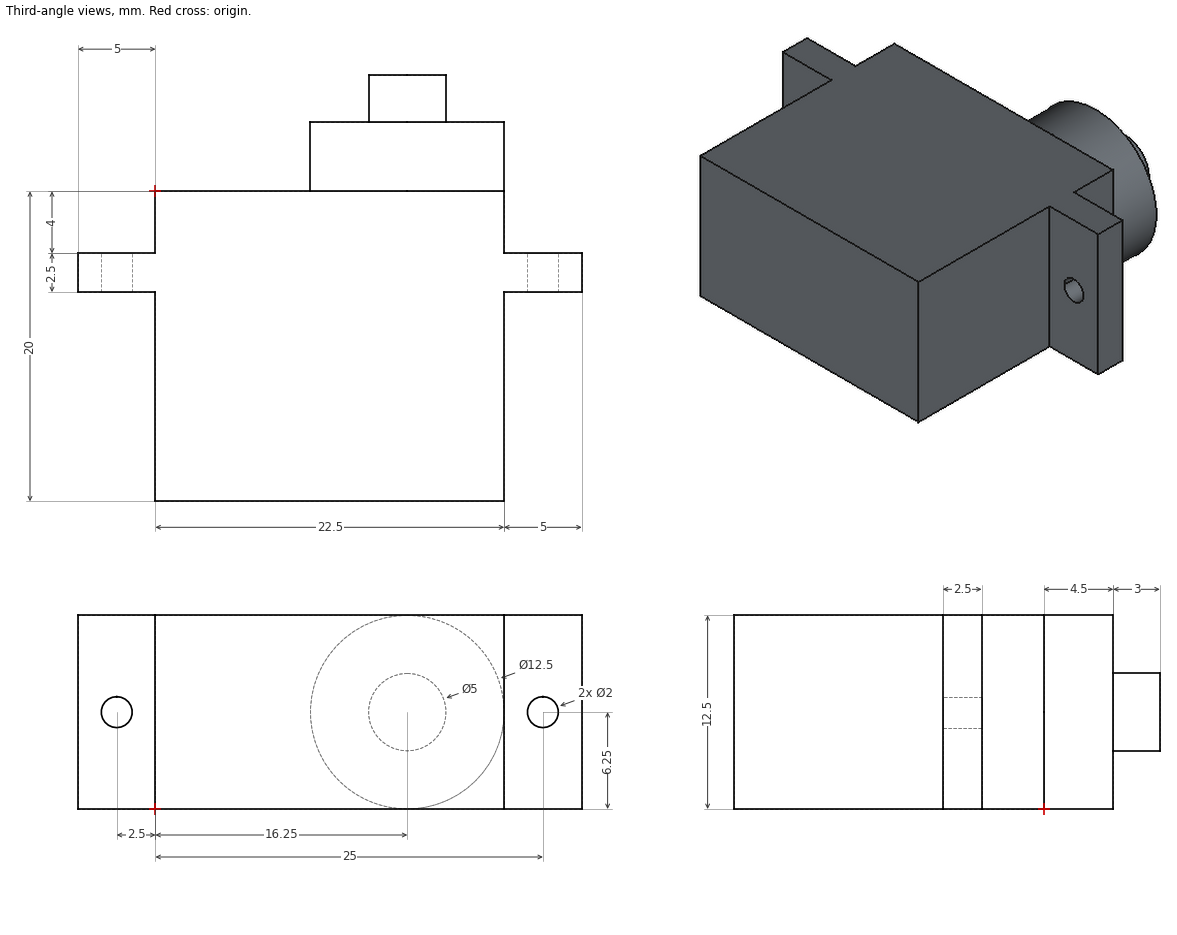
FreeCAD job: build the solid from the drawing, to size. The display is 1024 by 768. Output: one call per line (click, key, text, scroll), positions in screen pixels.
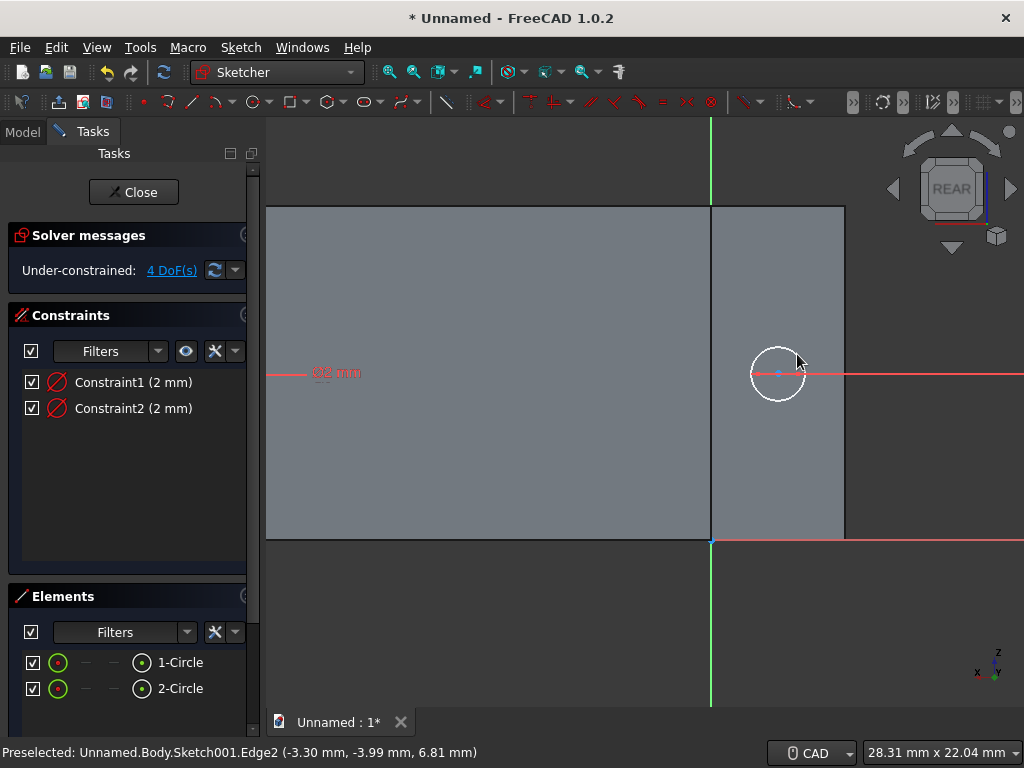
scroll(779, 374, down, 3)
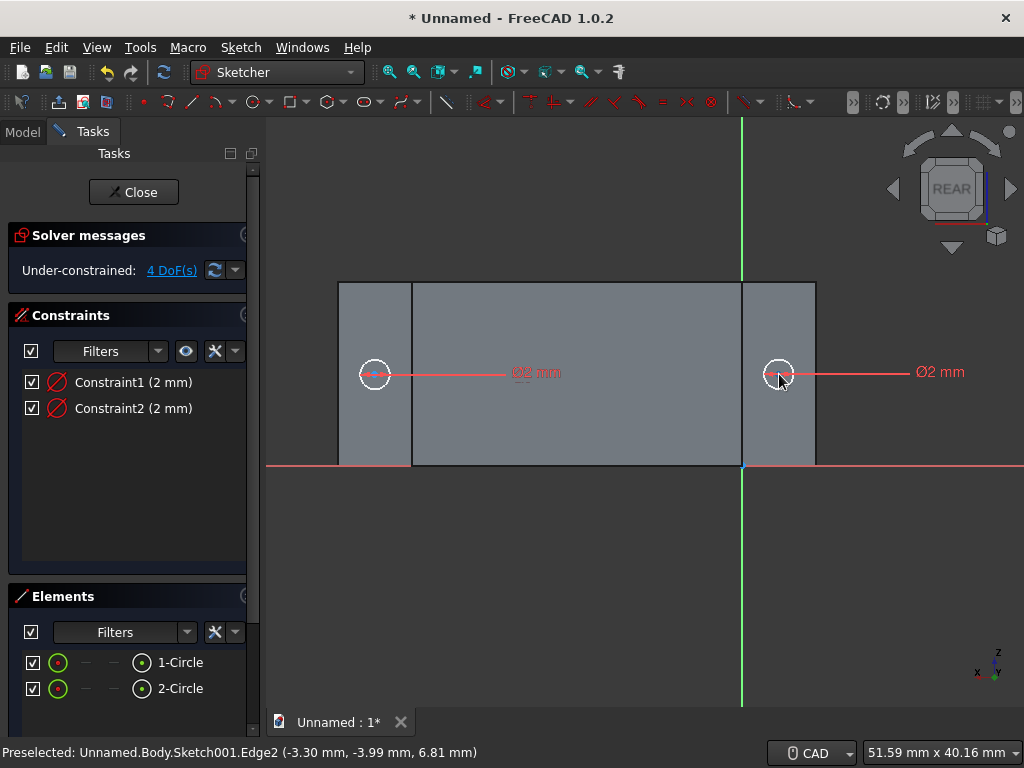
click(375, 375)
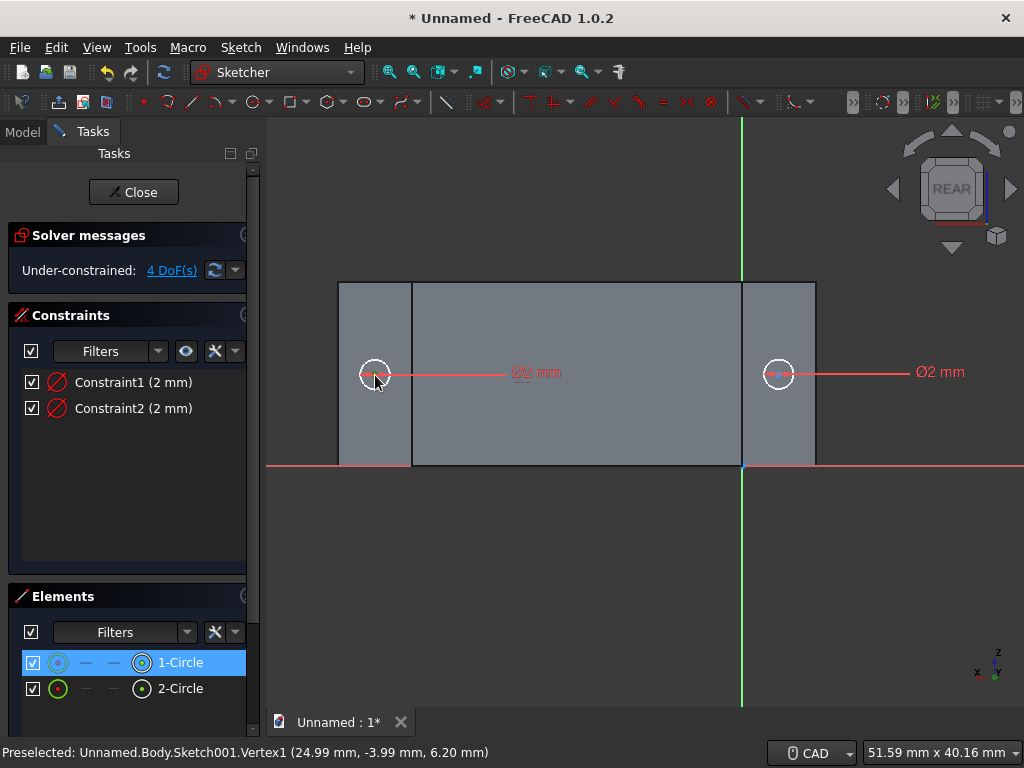
click(779, 374)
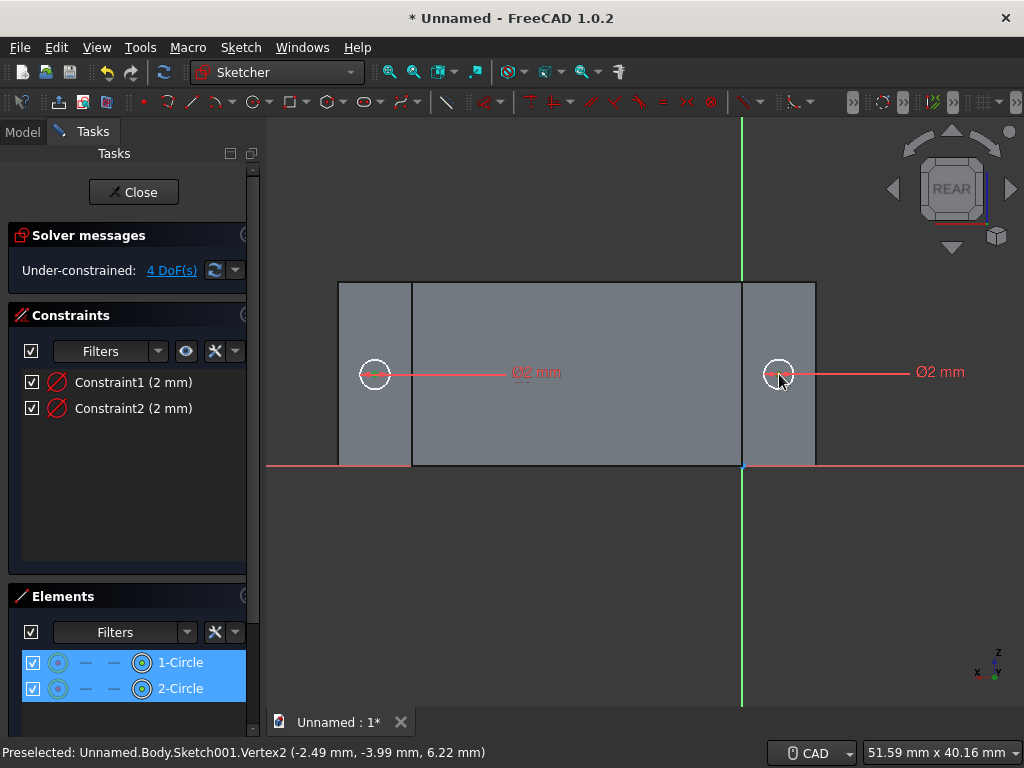
key(h)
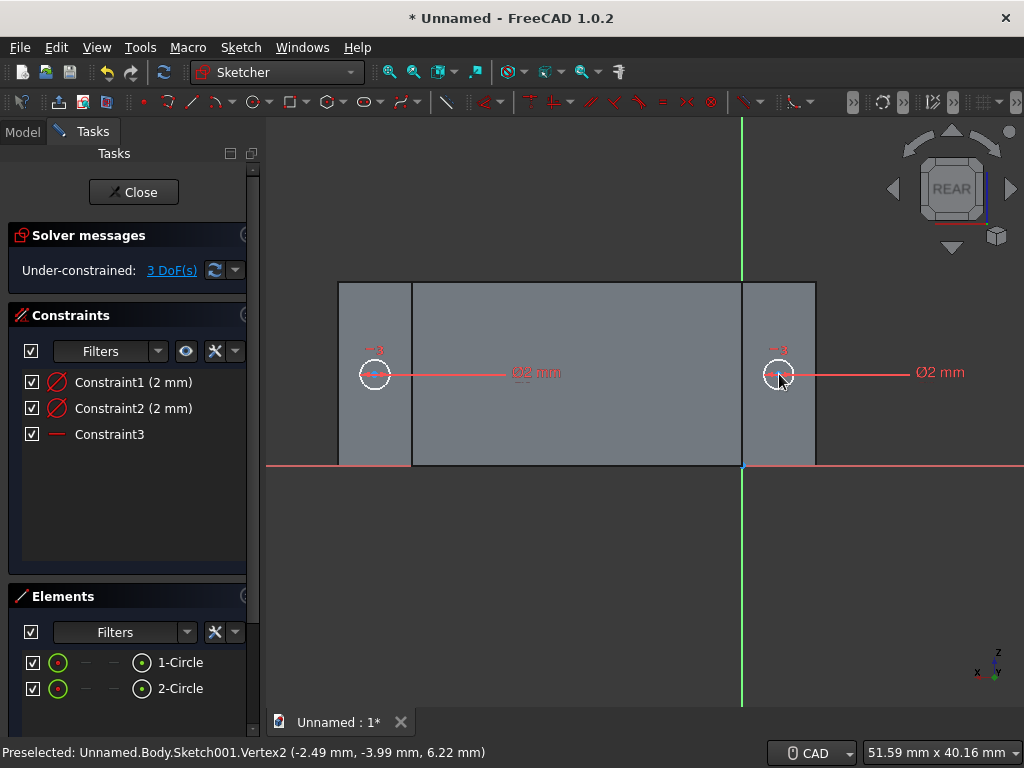
key(d)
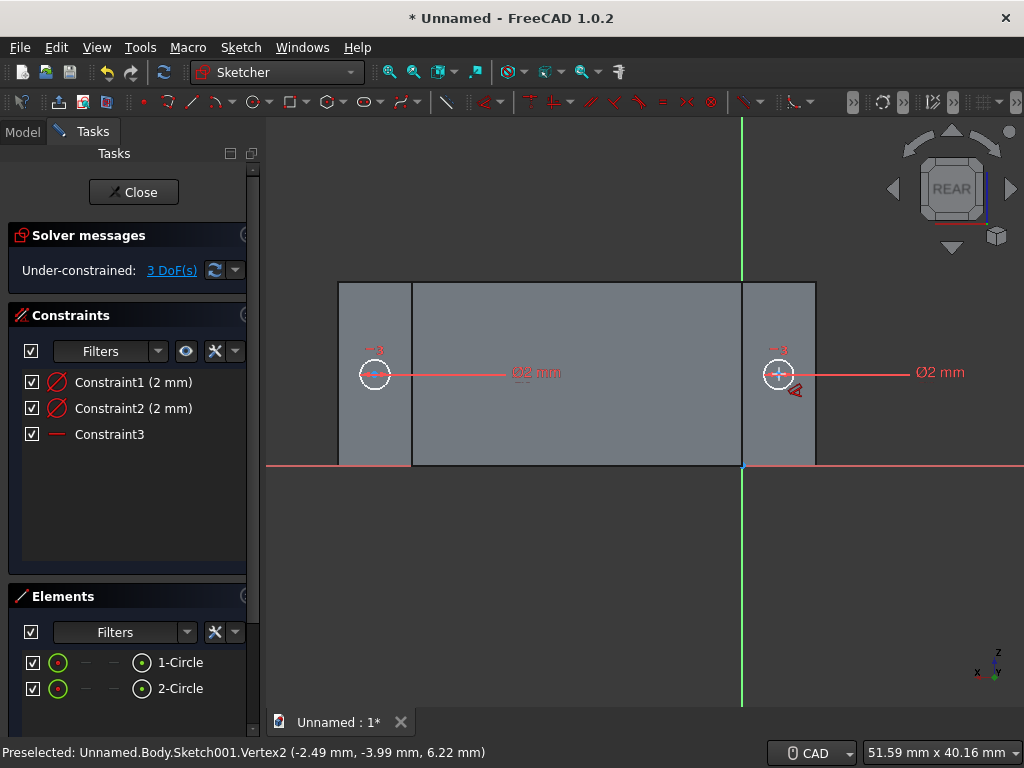
click(375, 375)
click(559, 500)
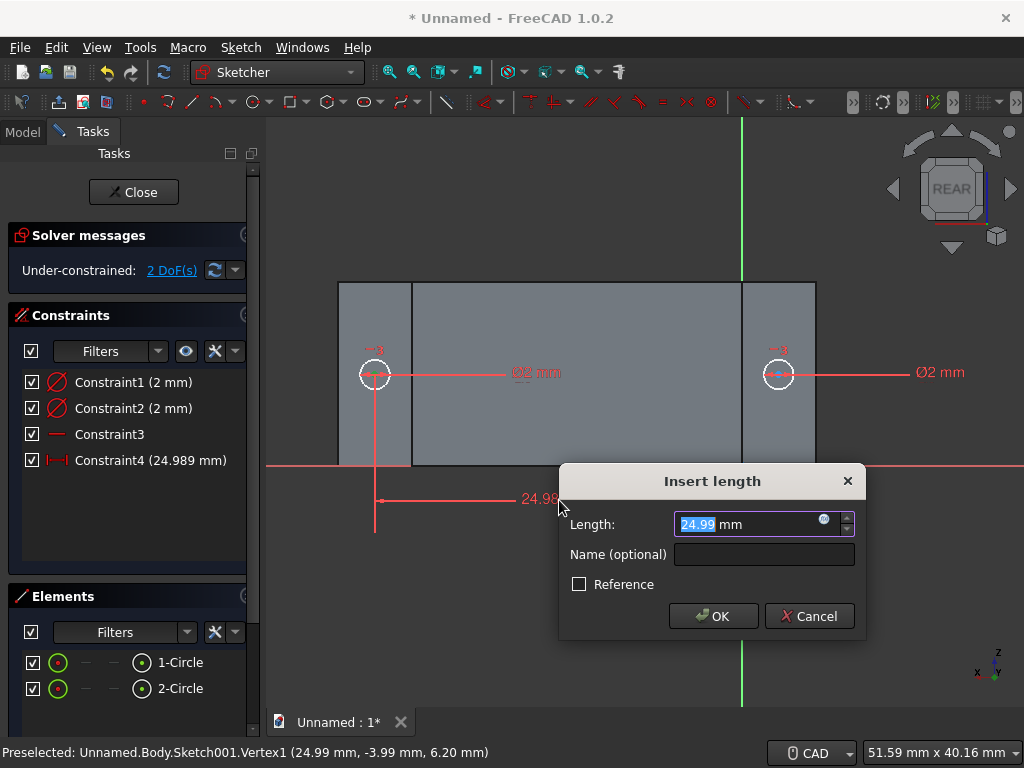
text(25)
key(Return)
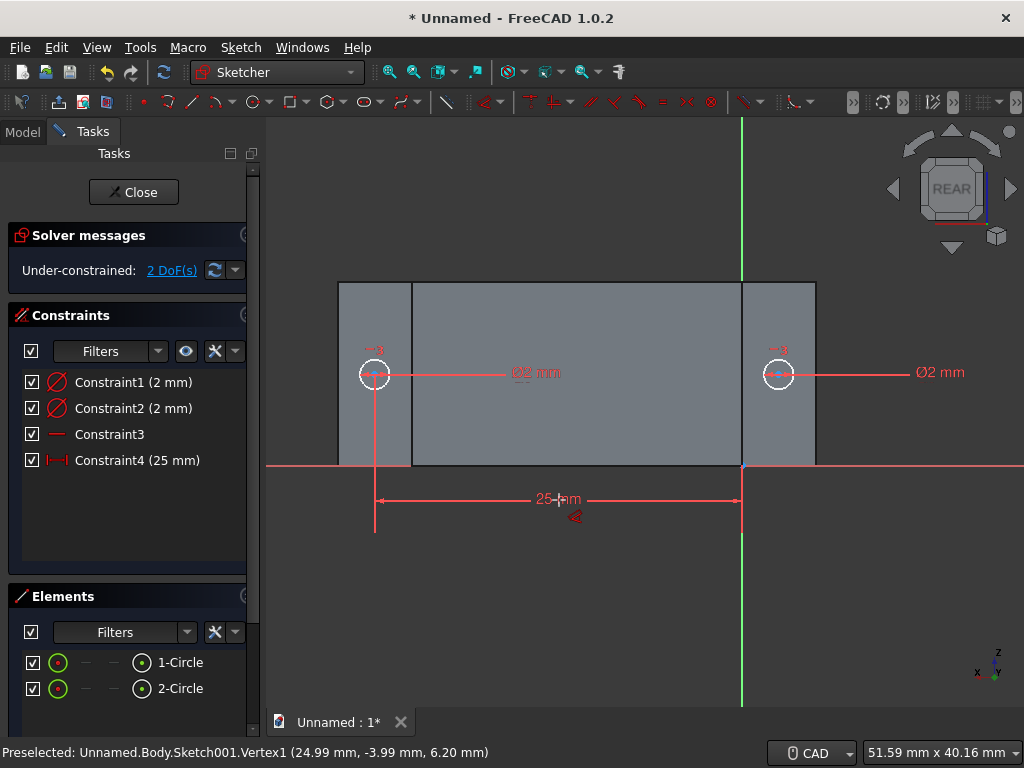
click(779, 375)
click(760, 500)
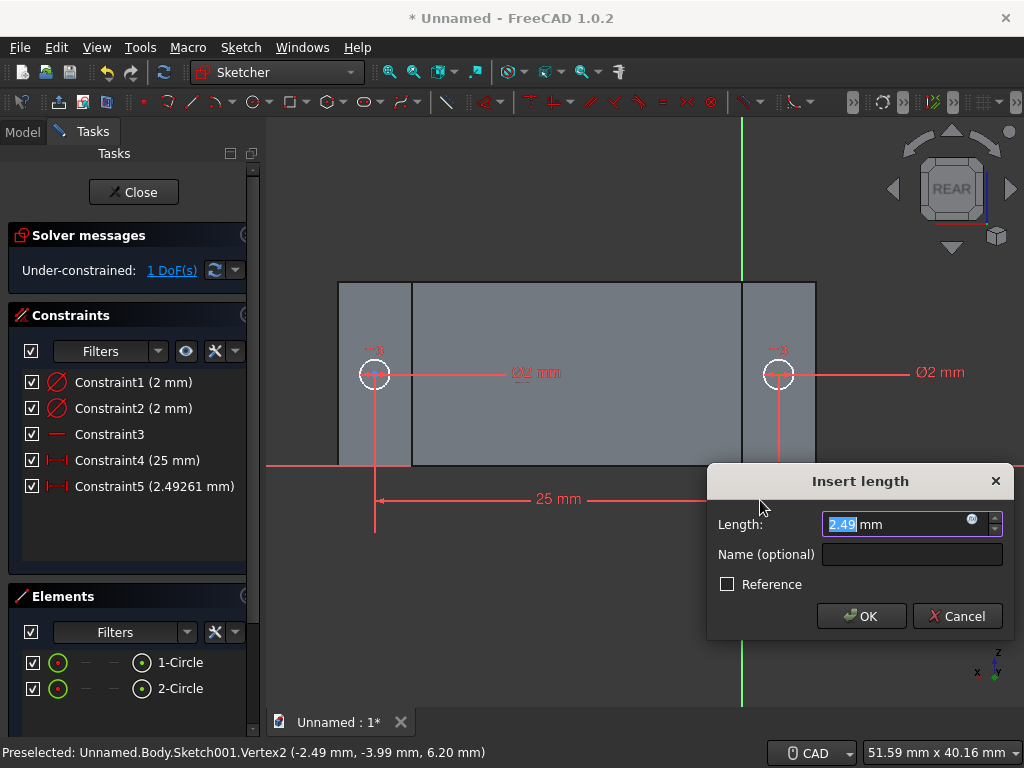
text(2.5)
key(Return)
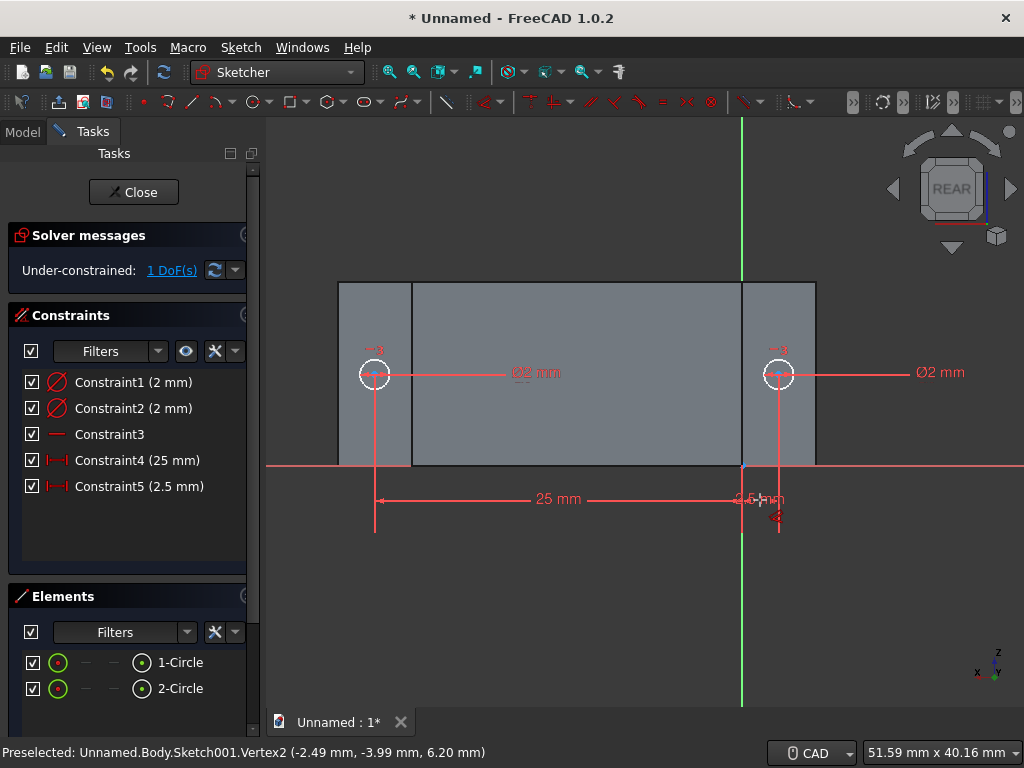
click(375, 375)
click(341, 420)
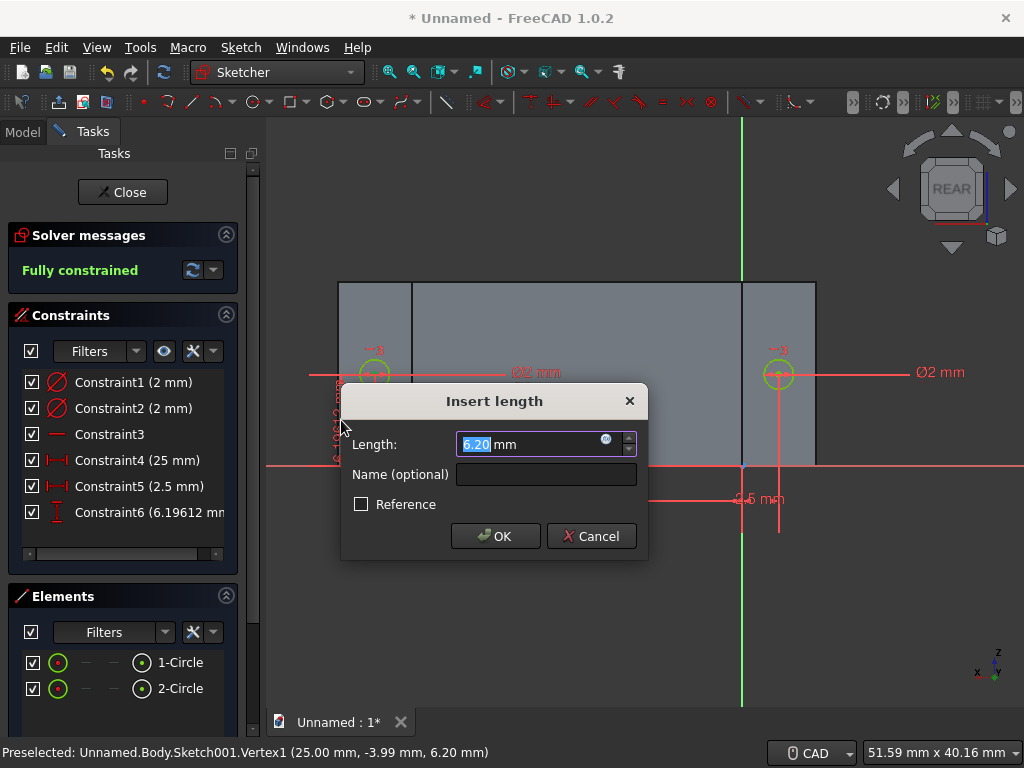
text(6.25)
key(Return)
key(Escape)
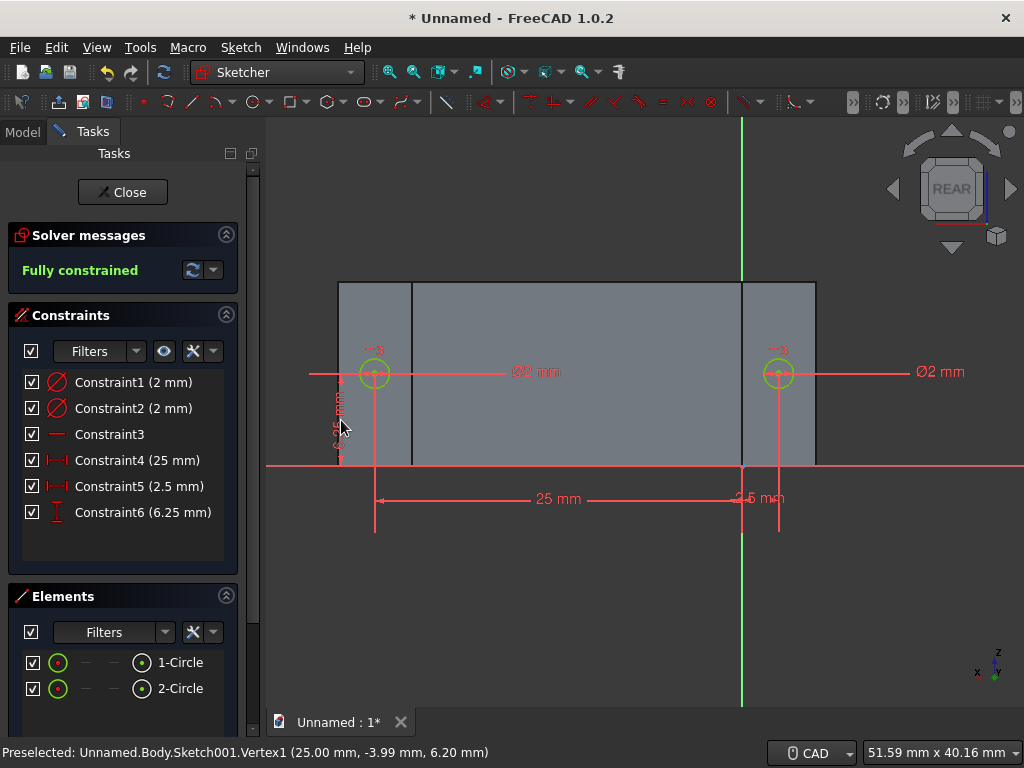
click(123, 192)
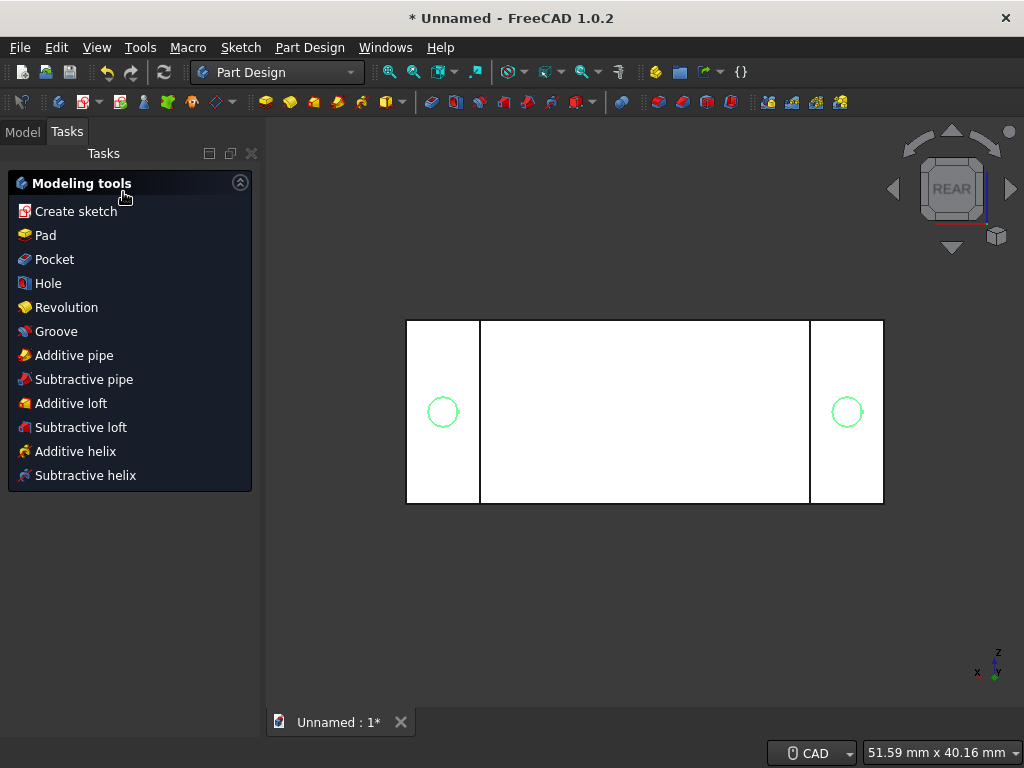
click(432, 102)